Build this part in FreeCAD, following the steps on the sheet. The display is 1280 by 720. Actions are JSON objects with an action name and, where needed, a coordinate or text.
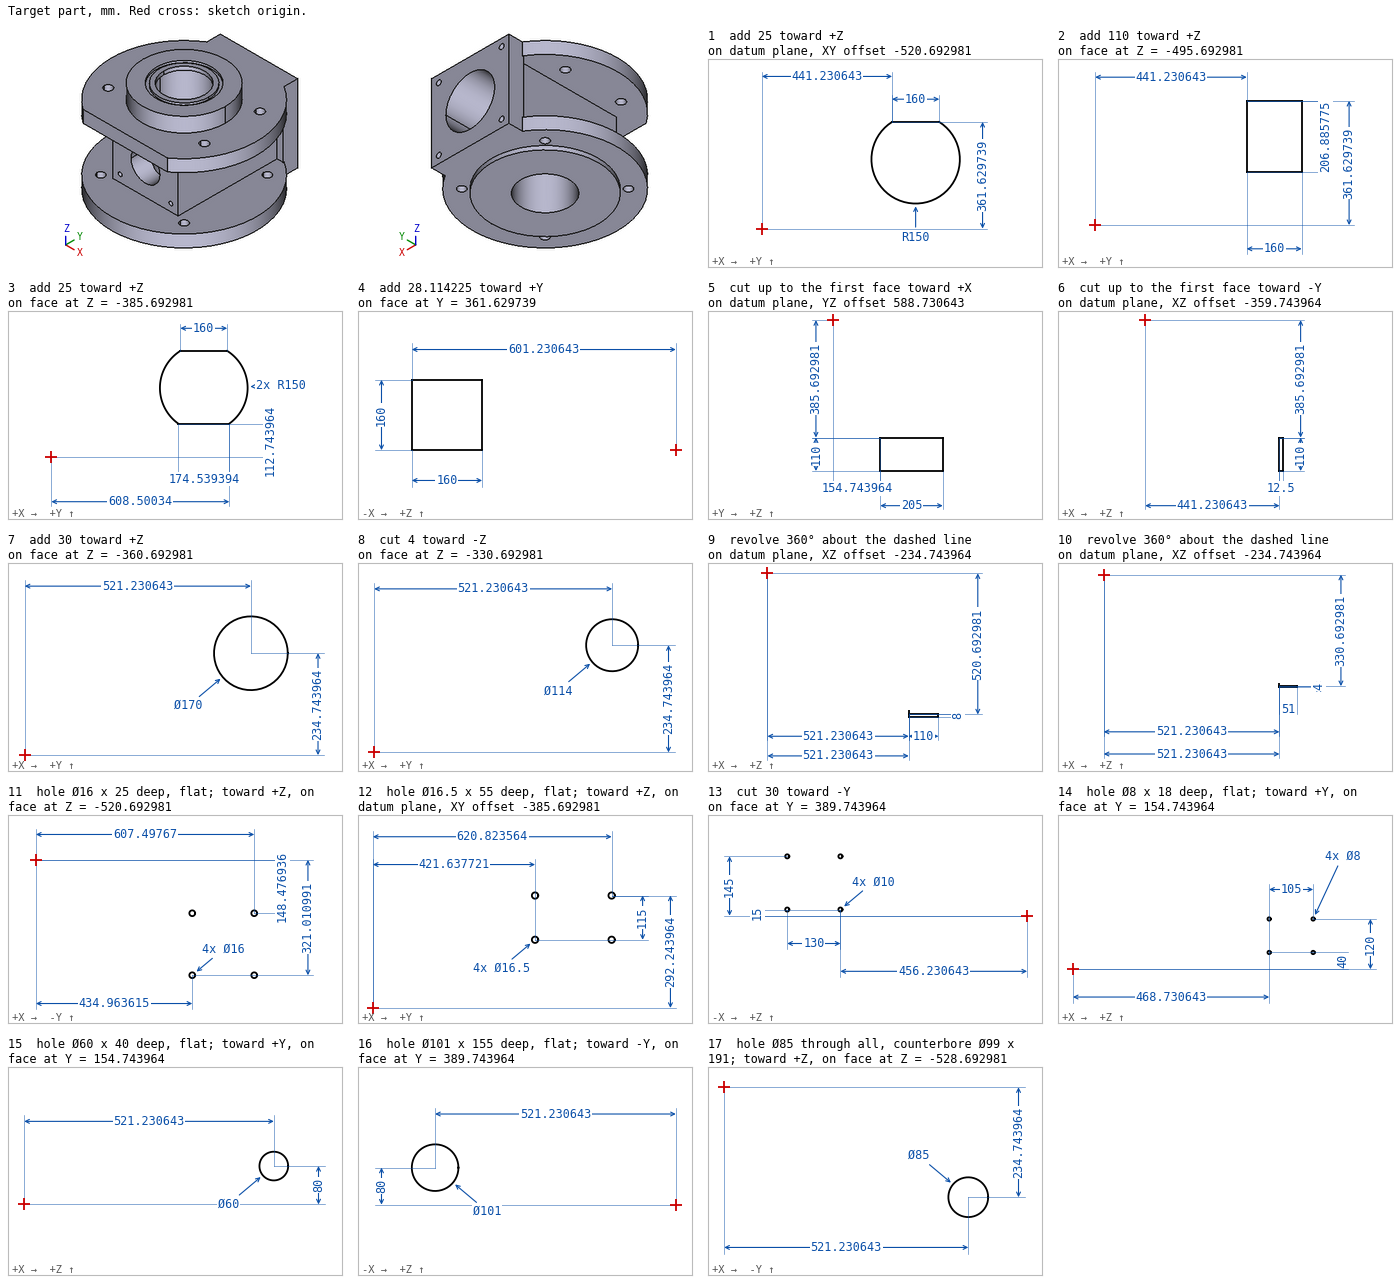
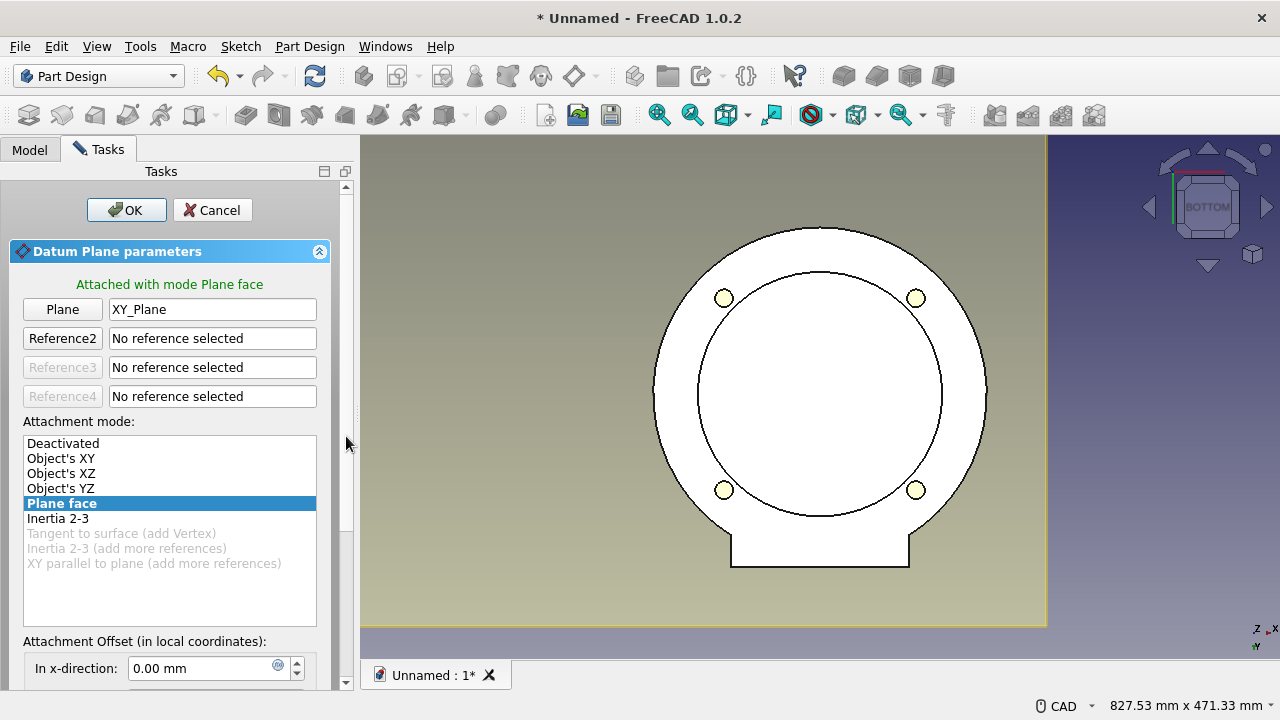
{"action": "left_click", "coordinate": [127, 210]}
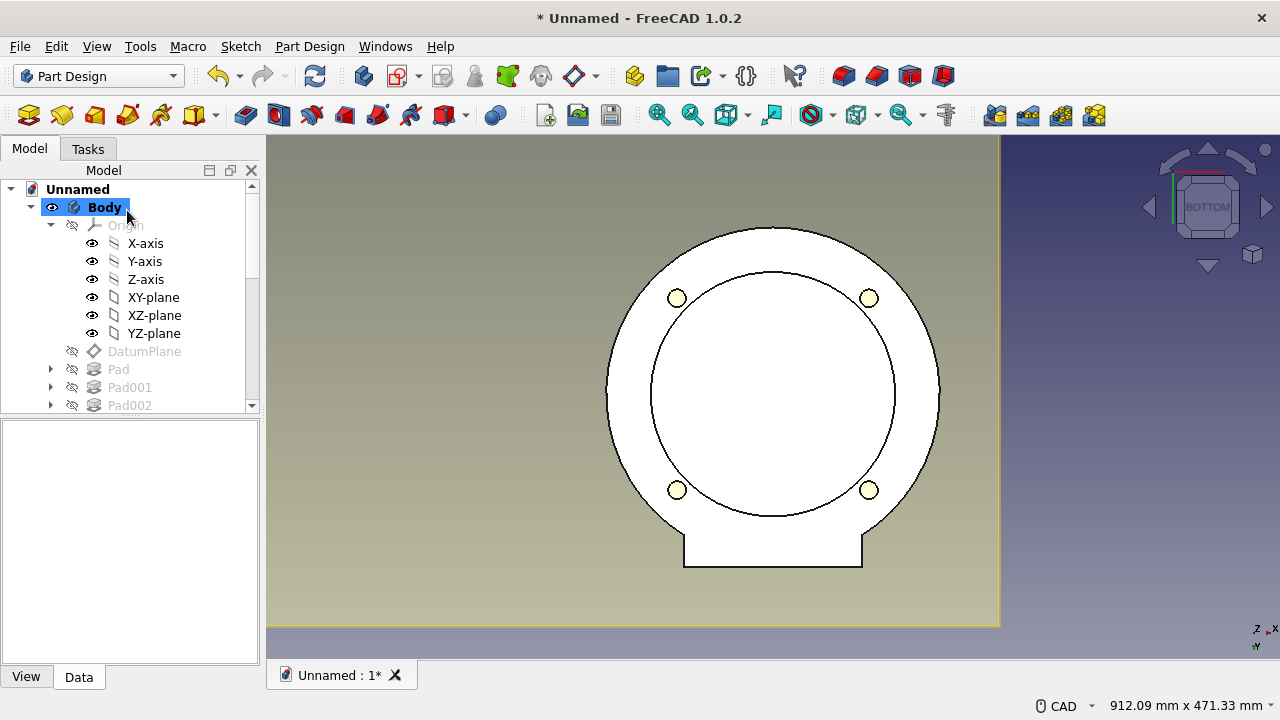
{"action": "scroll", "coordinate": [101, 293], "scroll_direction": "down", "scroll_amount": 3}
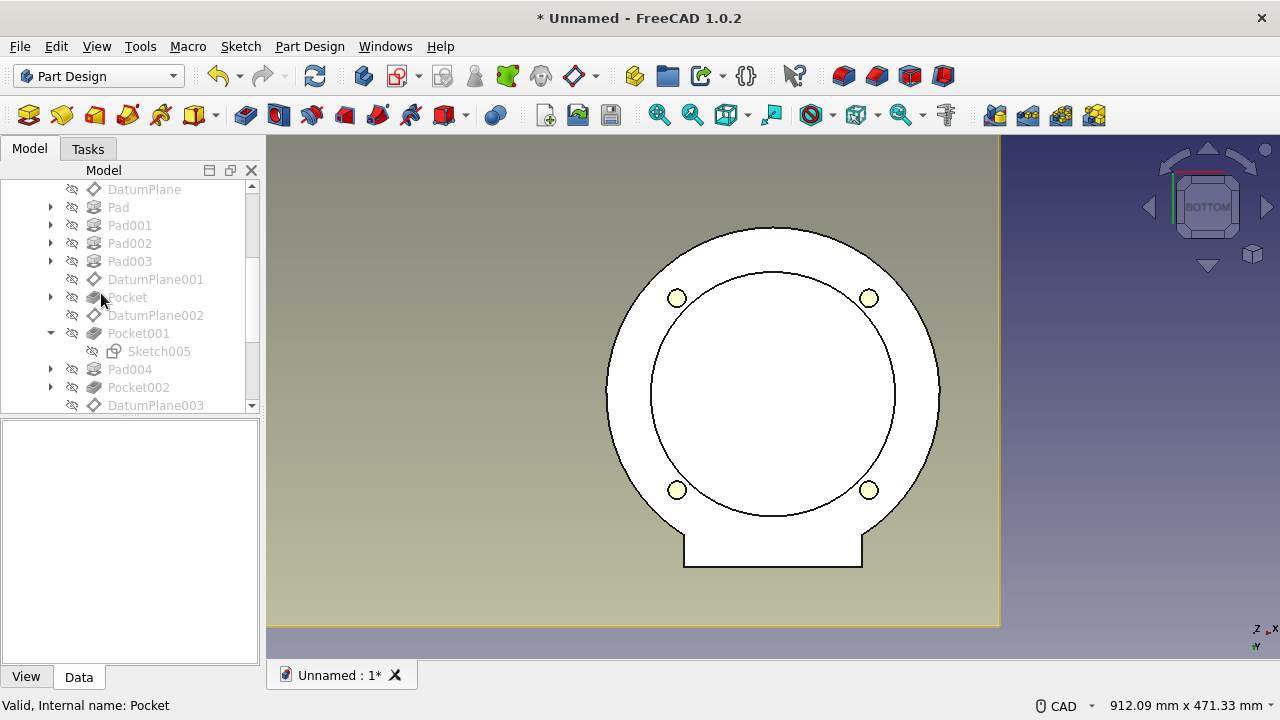
{"action": "scroll", "coordinate": [141, 293], "scroll_direction": "up", "scroll_amount": 15}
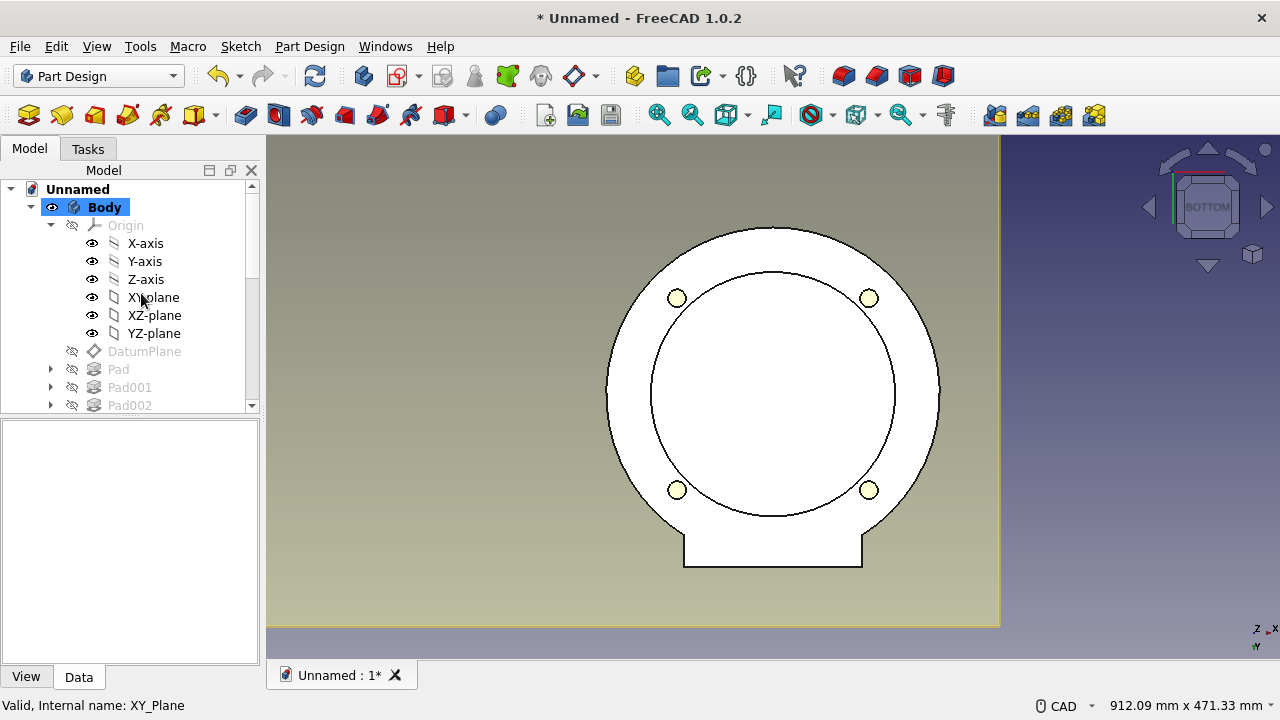
{"action": "scroll", "coordinate": [101, 293], "scroll_direction": "down", "scroll_amount": 6}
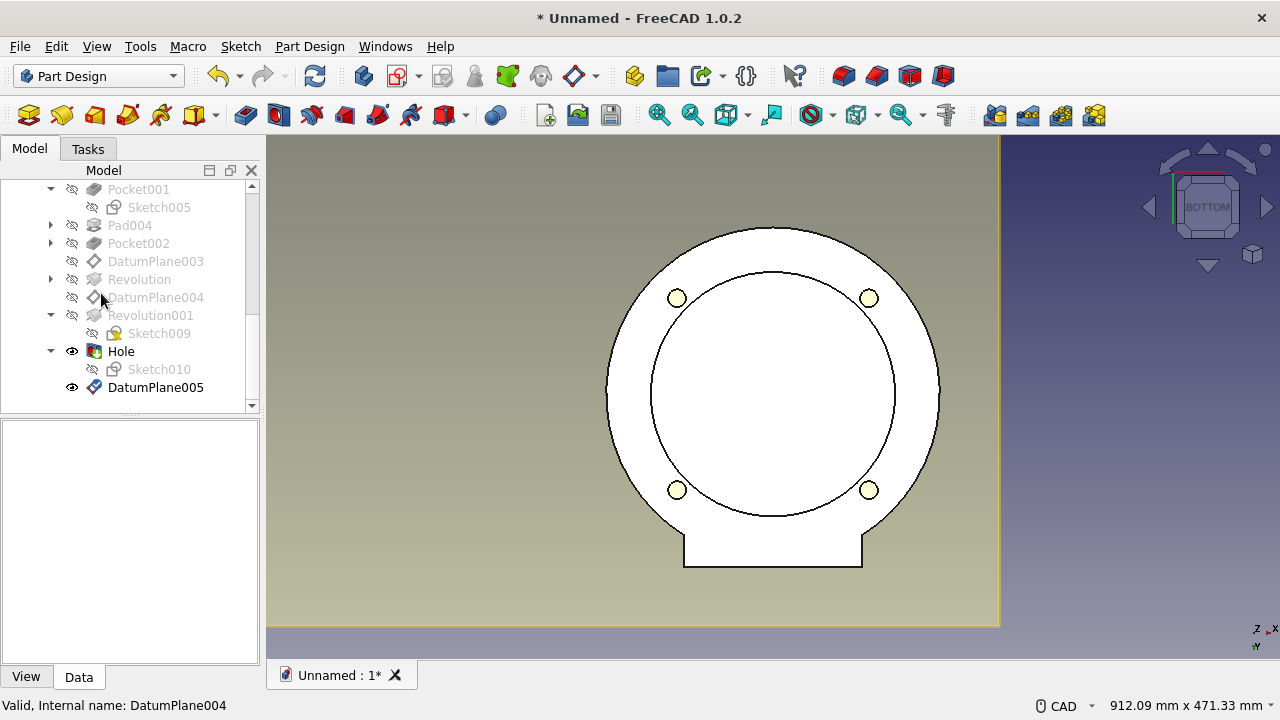
{"action": "left_click", "coordinate": [117, 387]}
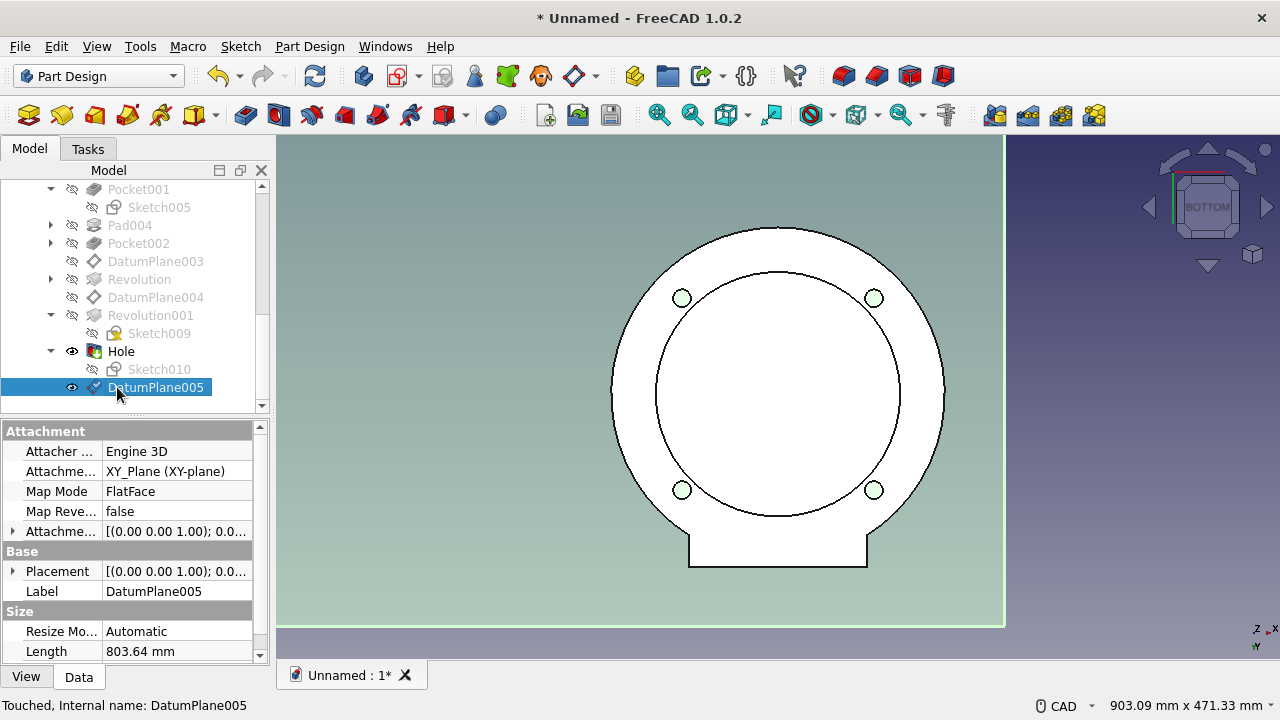
{"action": "left_click", "coordinate": [396, 76]}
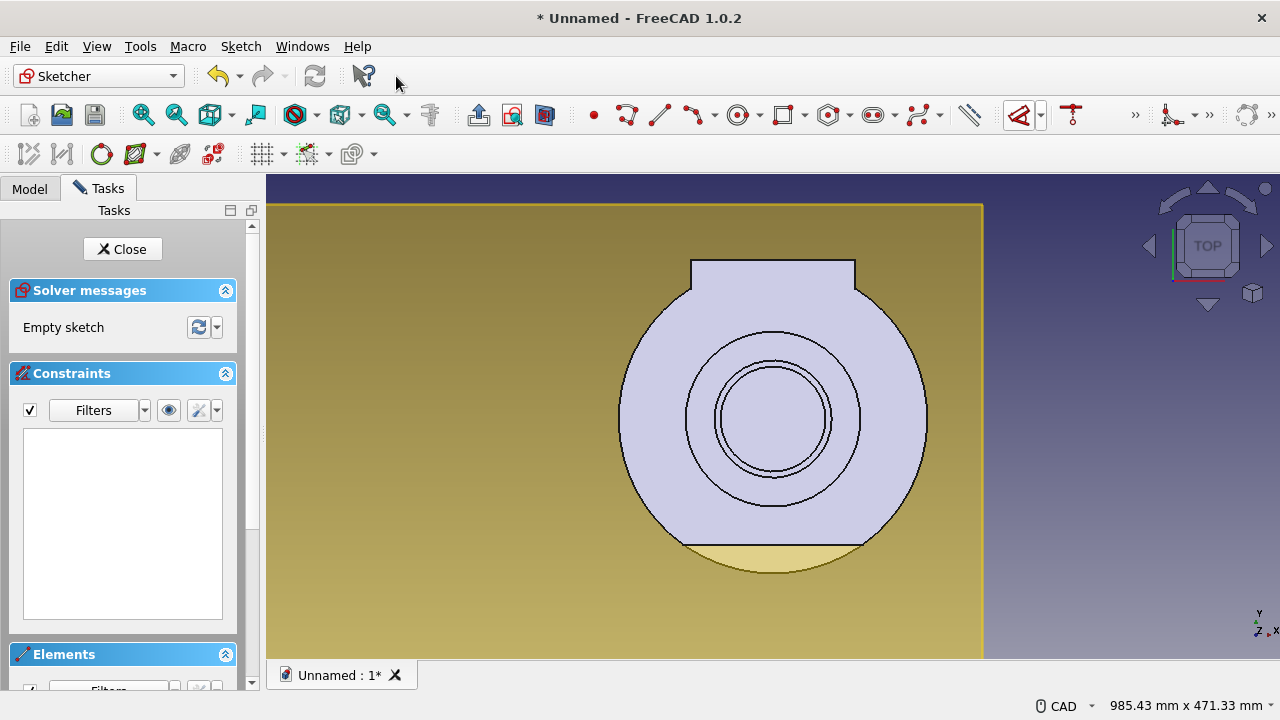
{"action": "left_click", "coordinate": [545, 116]}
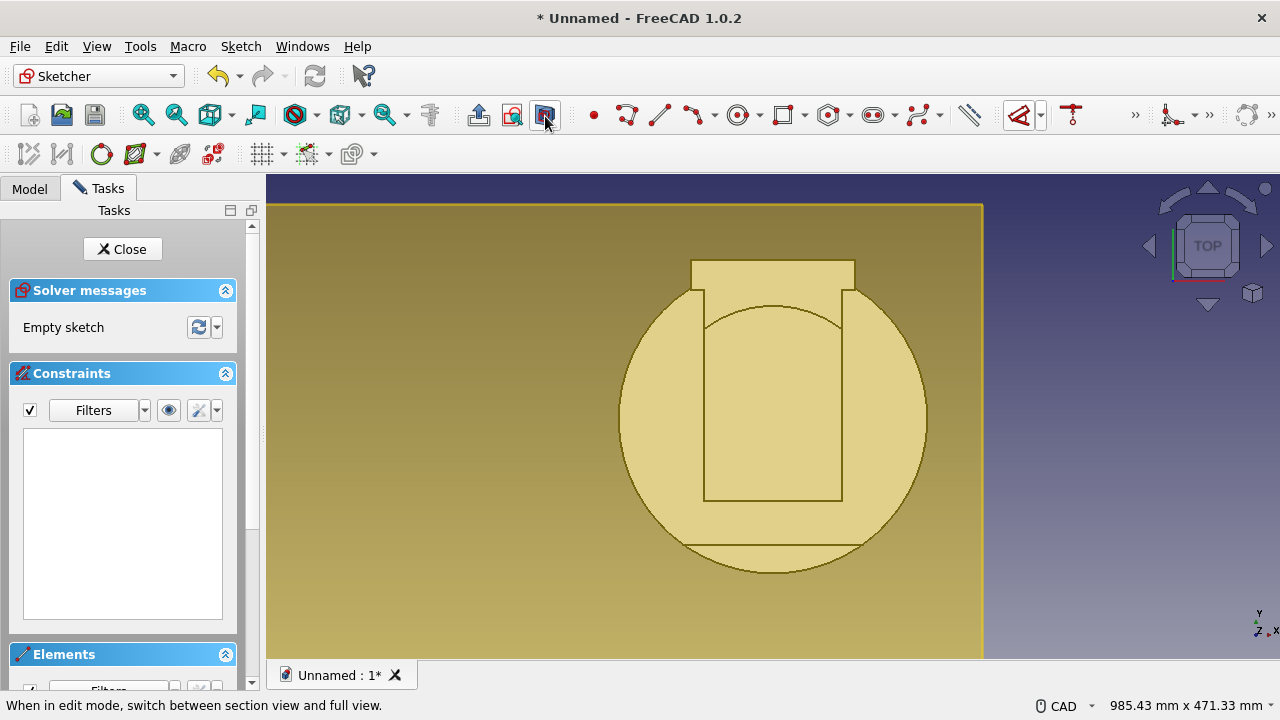
{"action": "scroll", "coordinate": [829, 421], "scroll_direction": "up", "scroll_amount": 4}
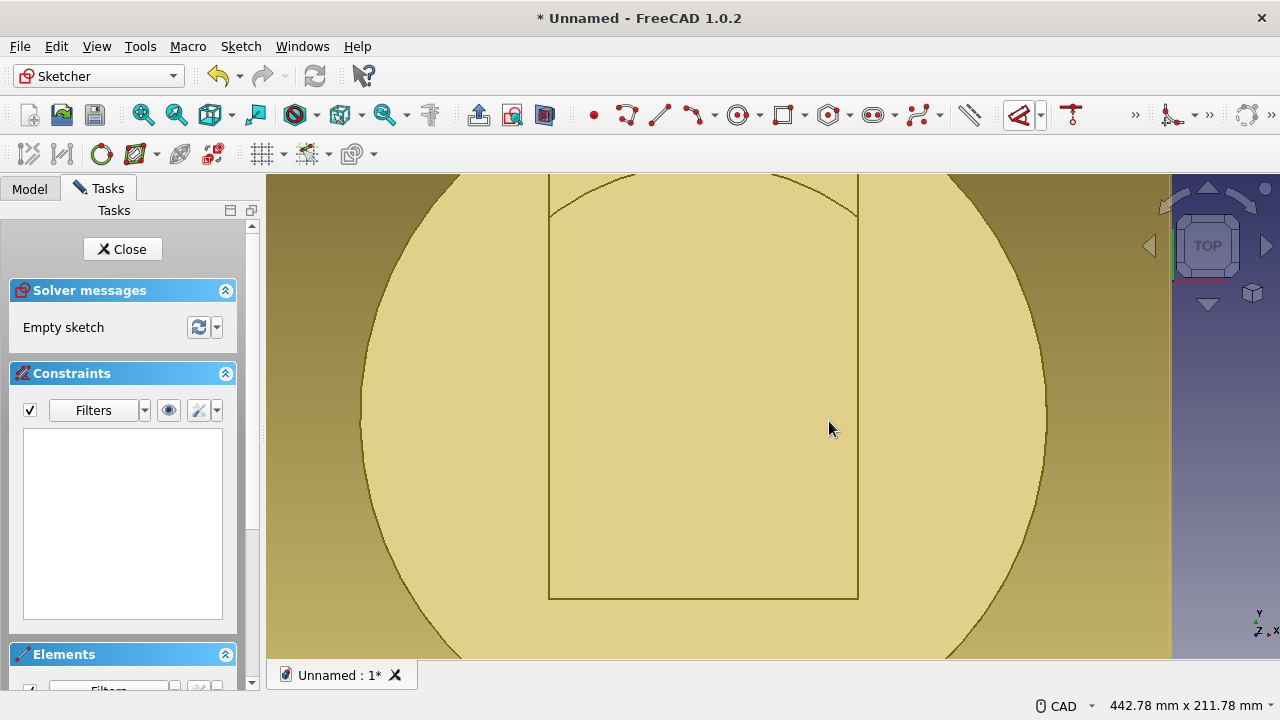
{"action": "left_click", "coordinate": [738, 116]}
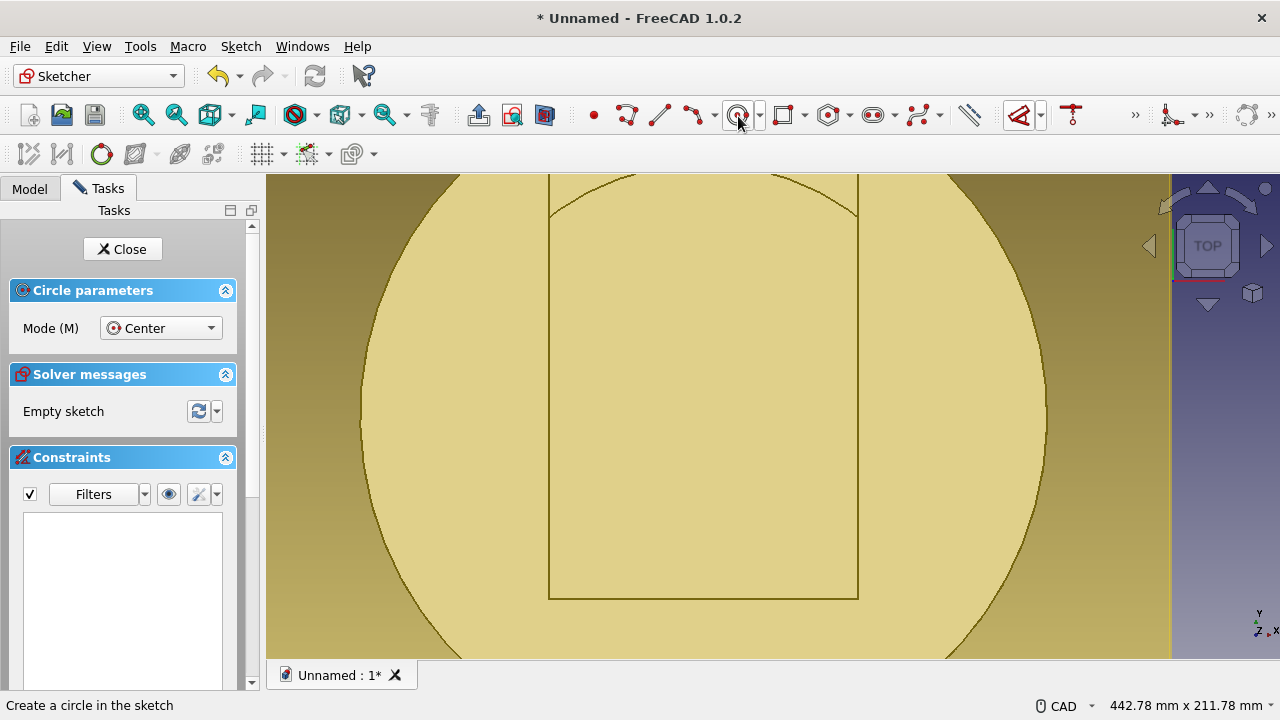
{"action": "left_click", "coordinate": [932, 284]}
{"action": "left_click", "coordinate": [945, 271]}